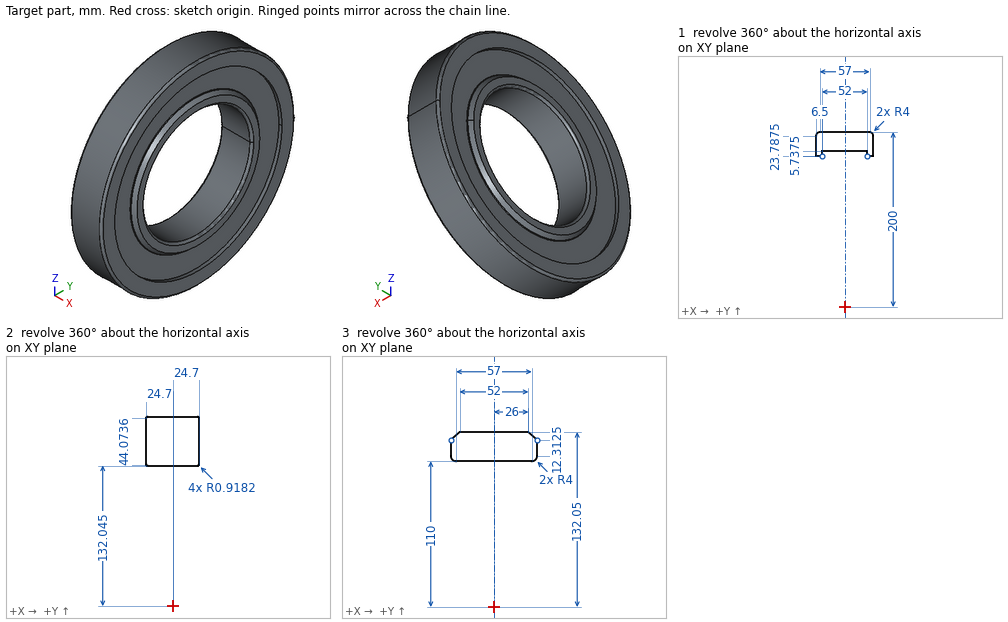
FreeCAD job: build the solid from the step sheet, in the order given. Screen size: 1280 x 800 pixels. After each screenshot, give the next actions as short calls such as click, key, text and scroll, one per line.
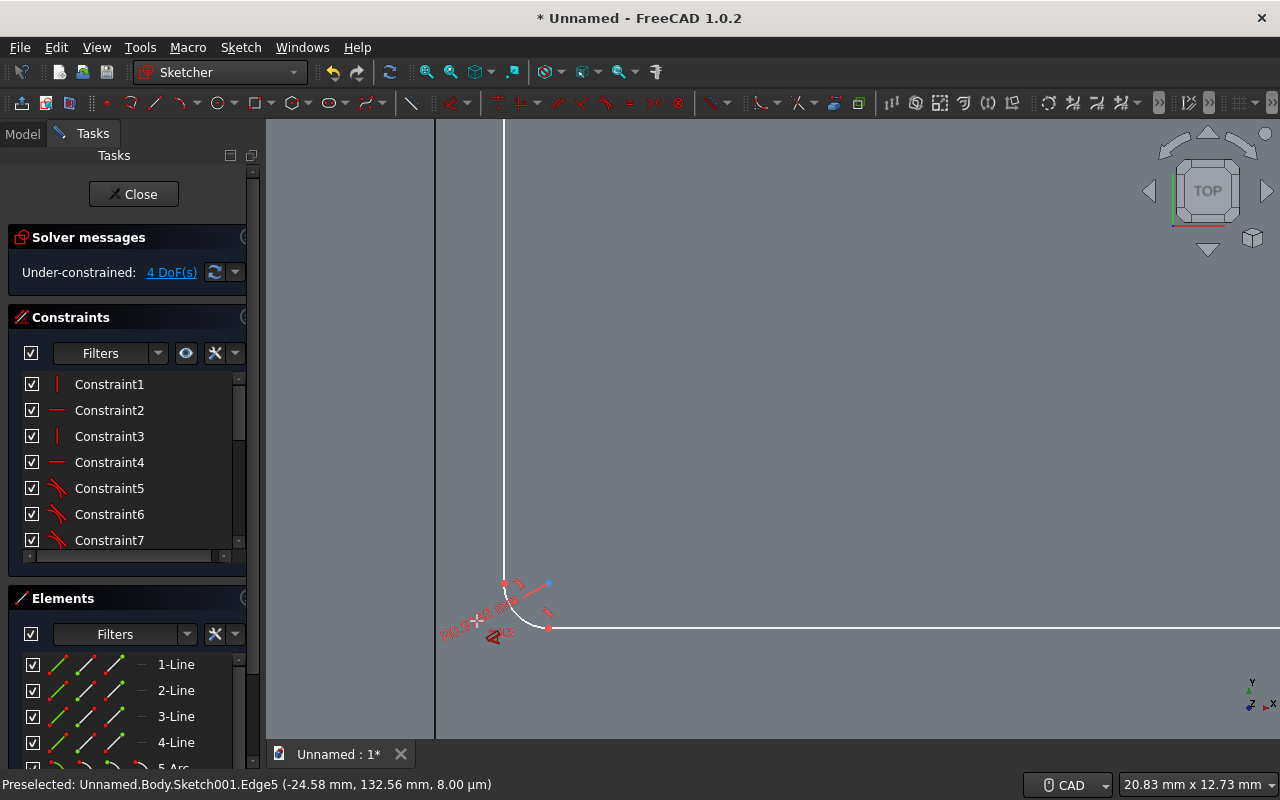
scroll(507, 611, down, 9)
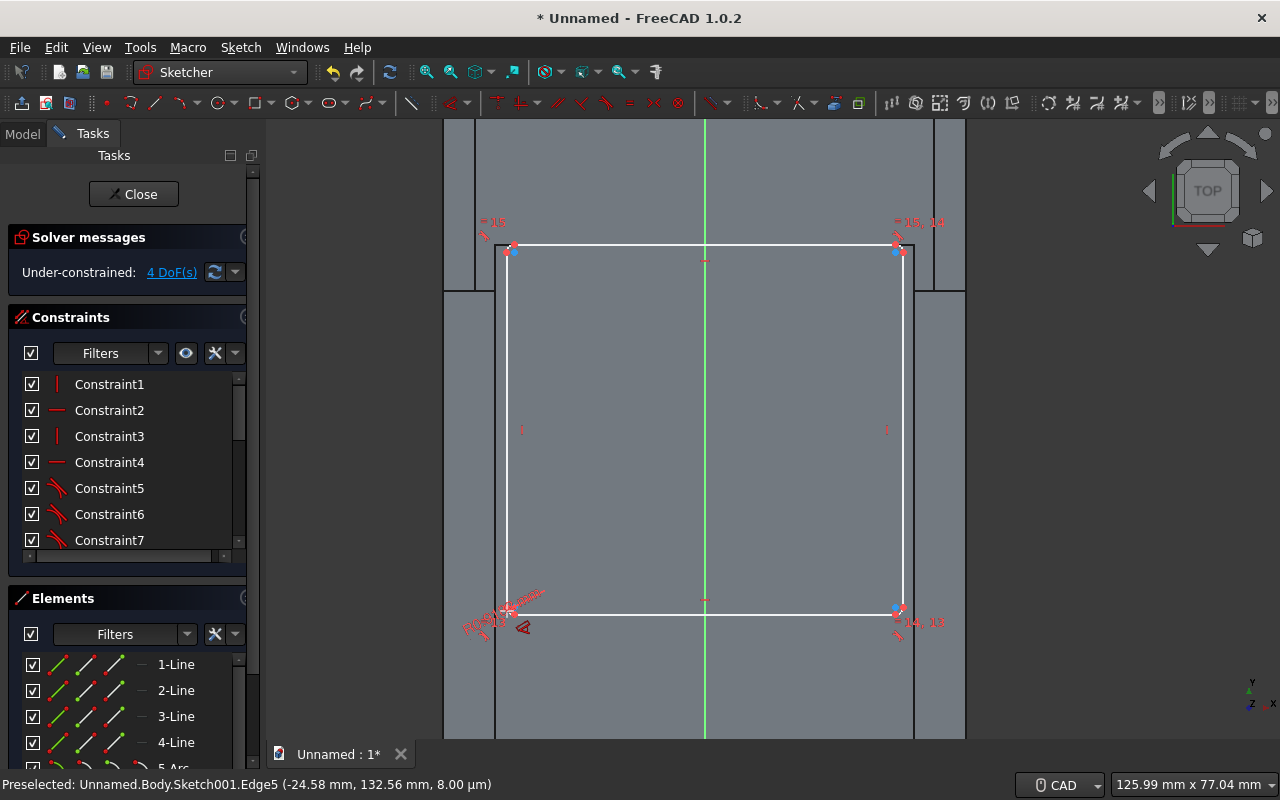
scroll(507, 252, up, 3)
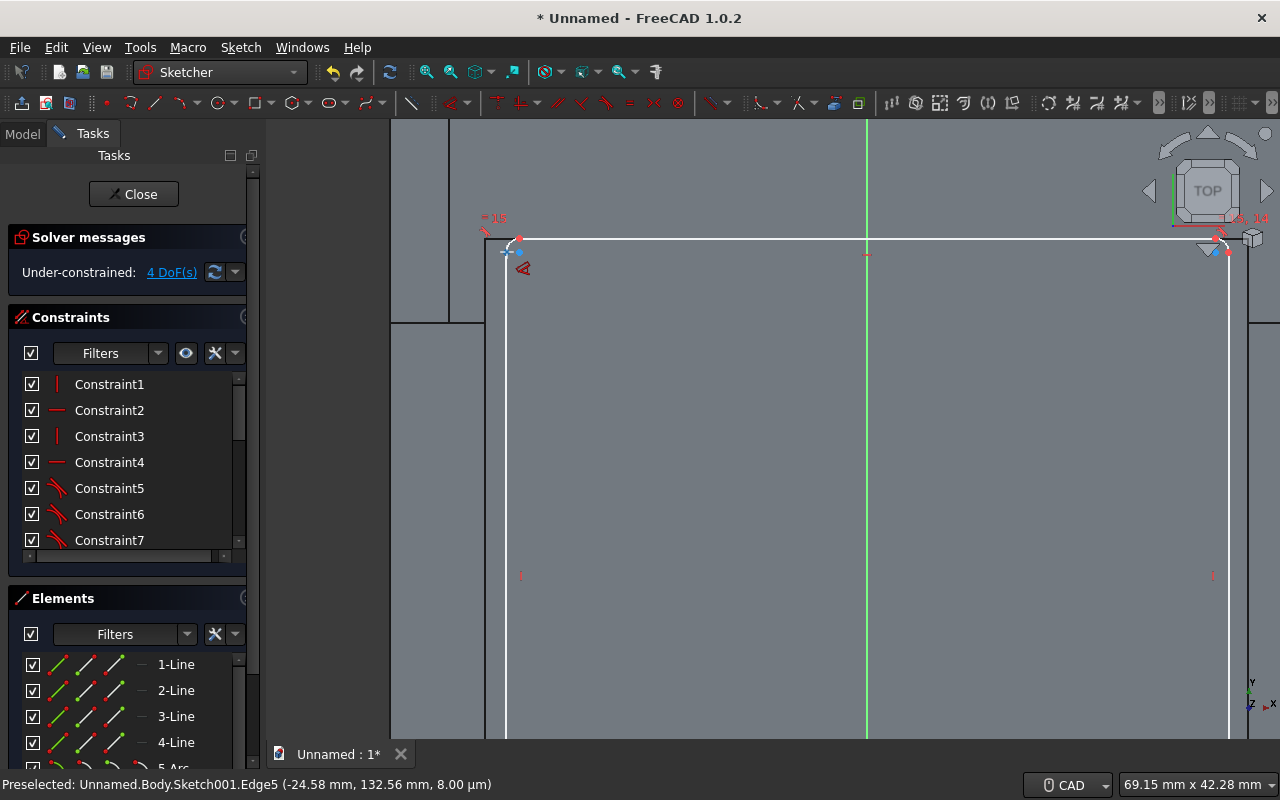
click(506, 252)
click(686, 218)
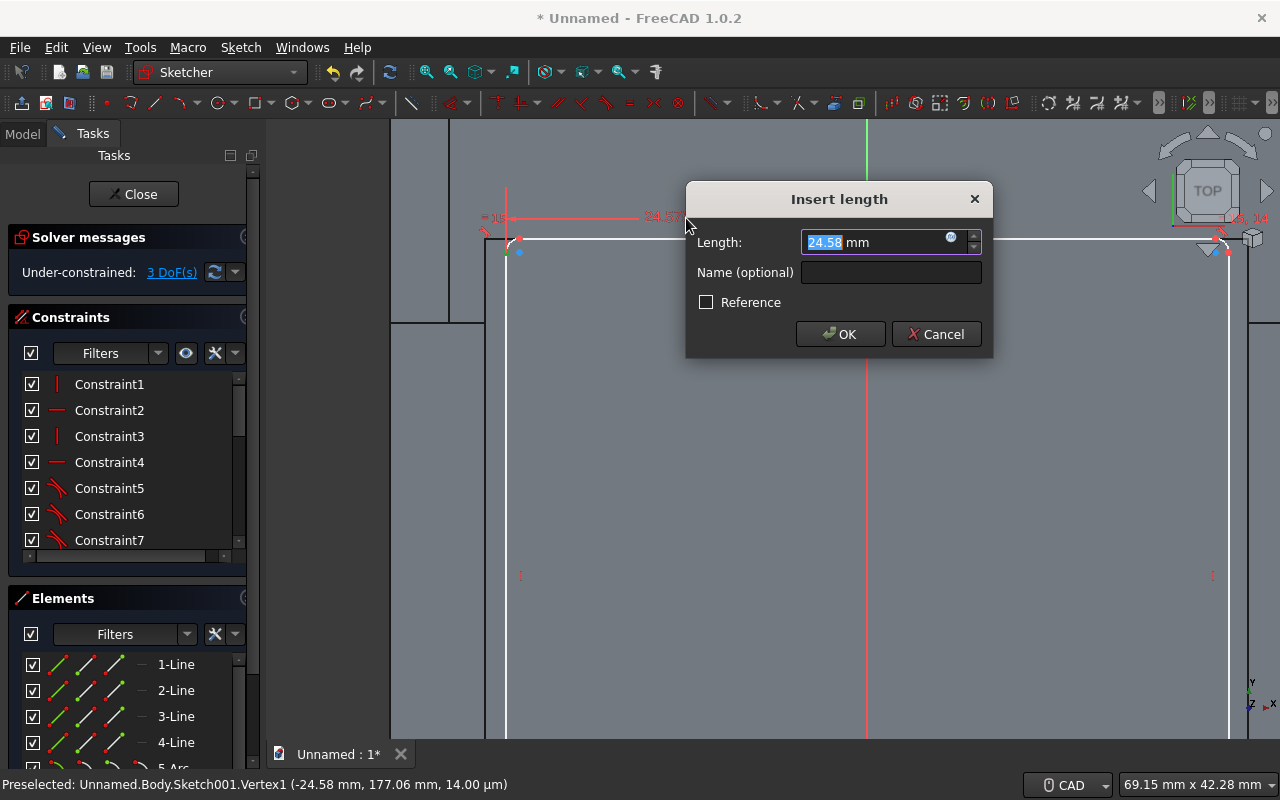
text(24.7)
key(Return)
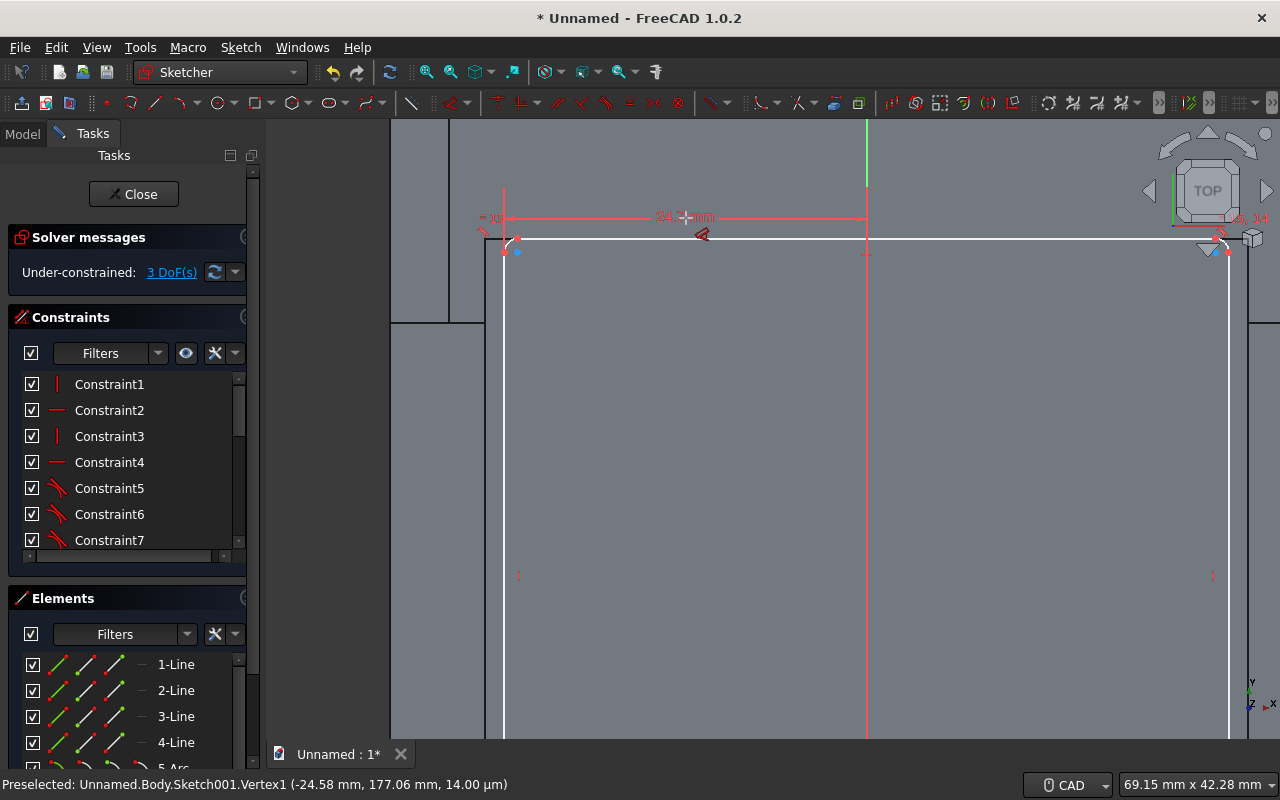
scroll(507, 251, down, 3)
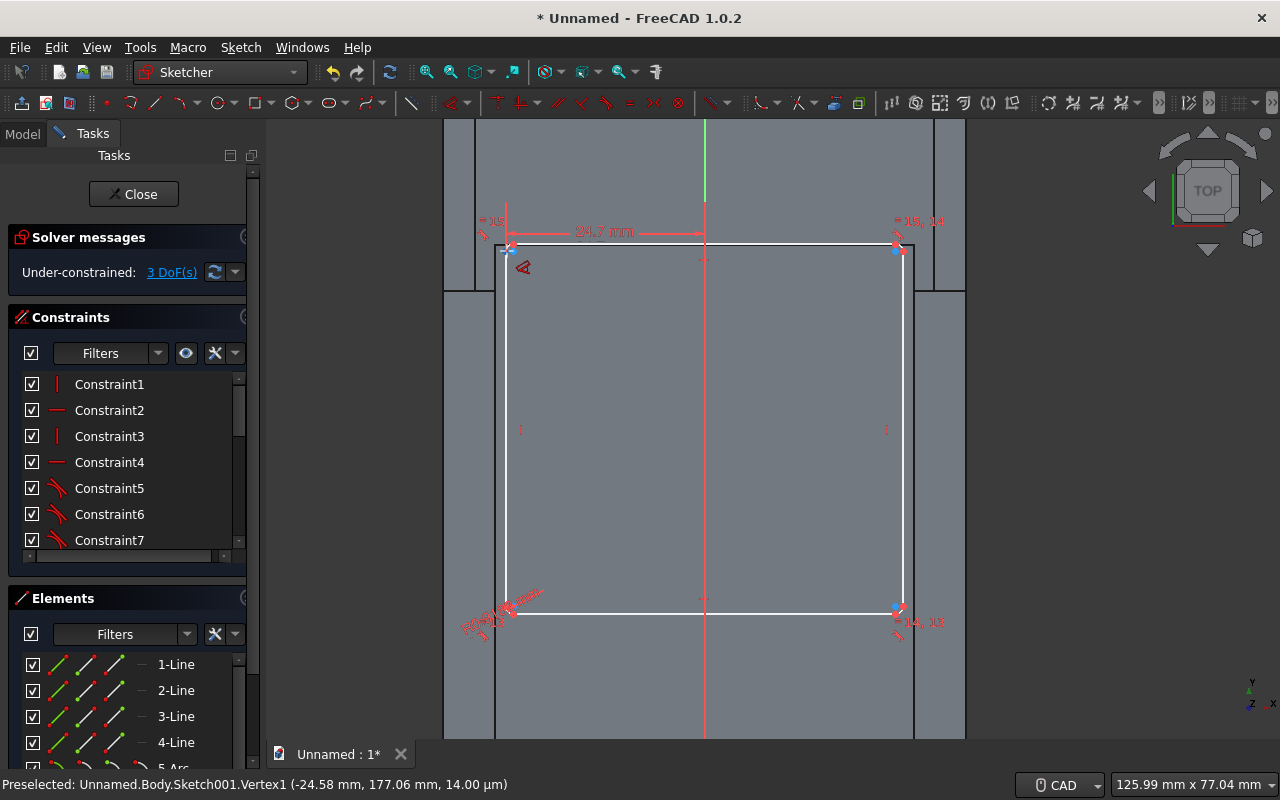
scroll(903, 607, up, 3)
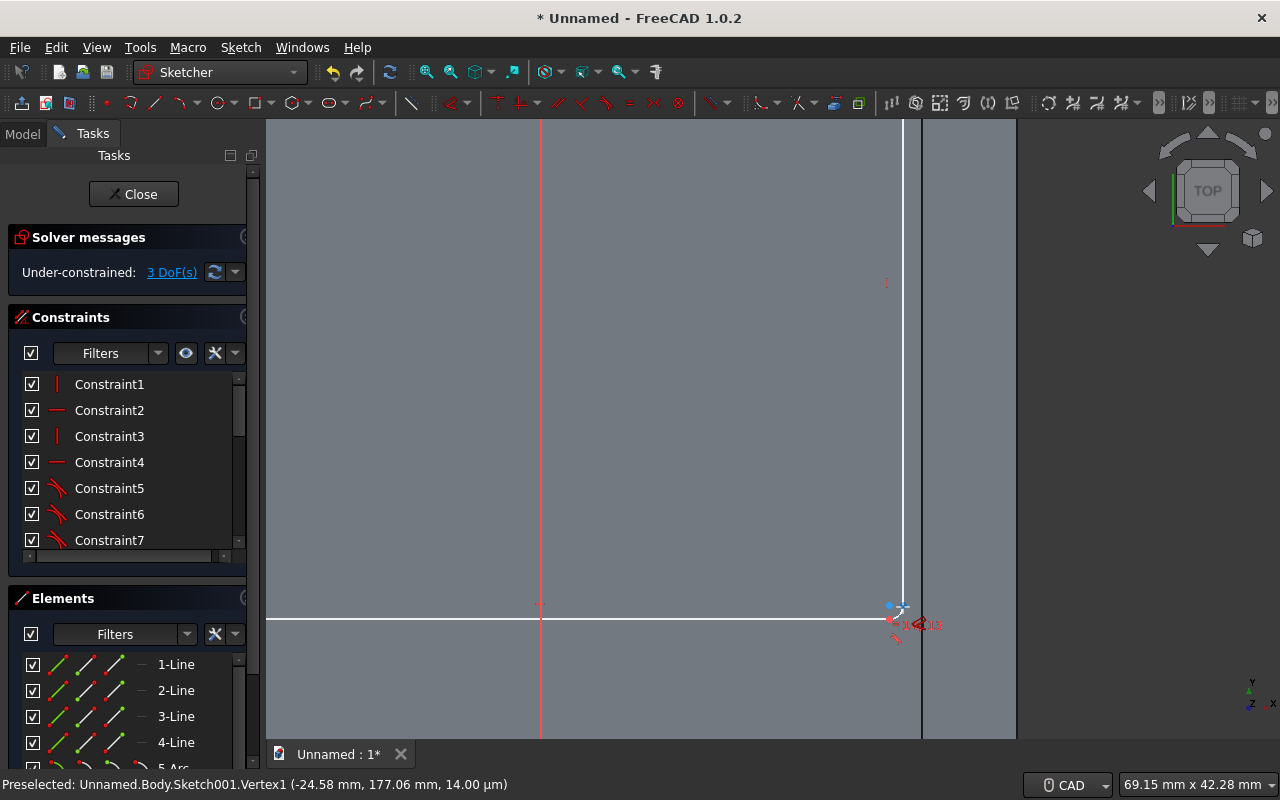
click(903, 606)
click(722, 572)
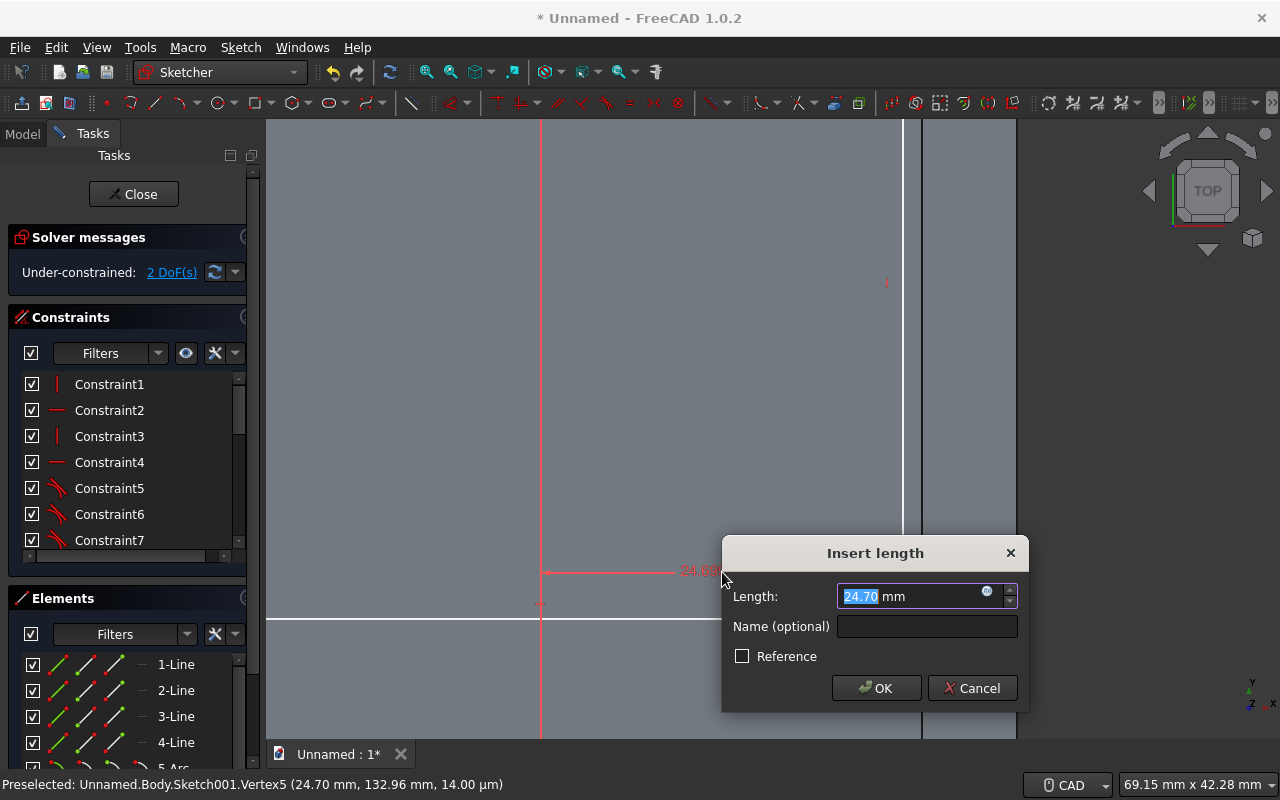
text(24.7)
key(Return)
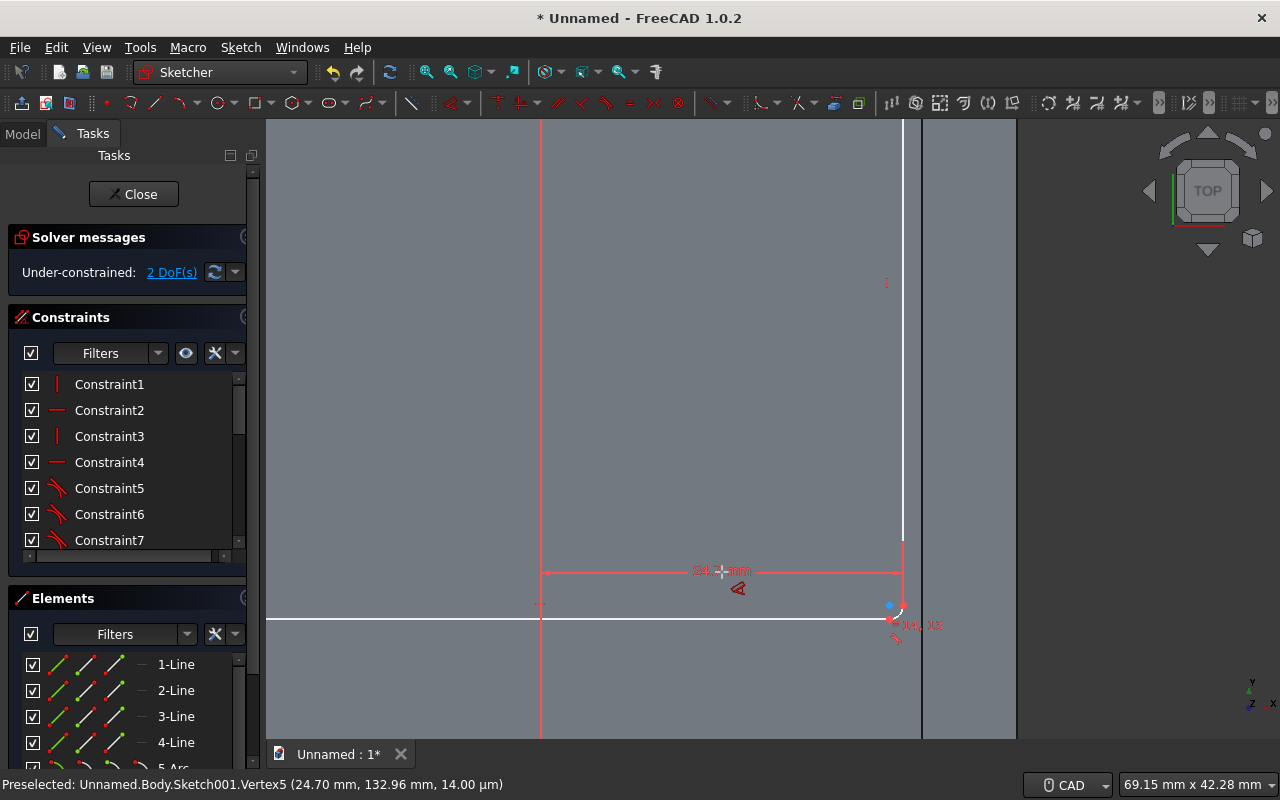
scroll(904, 607, down, 3)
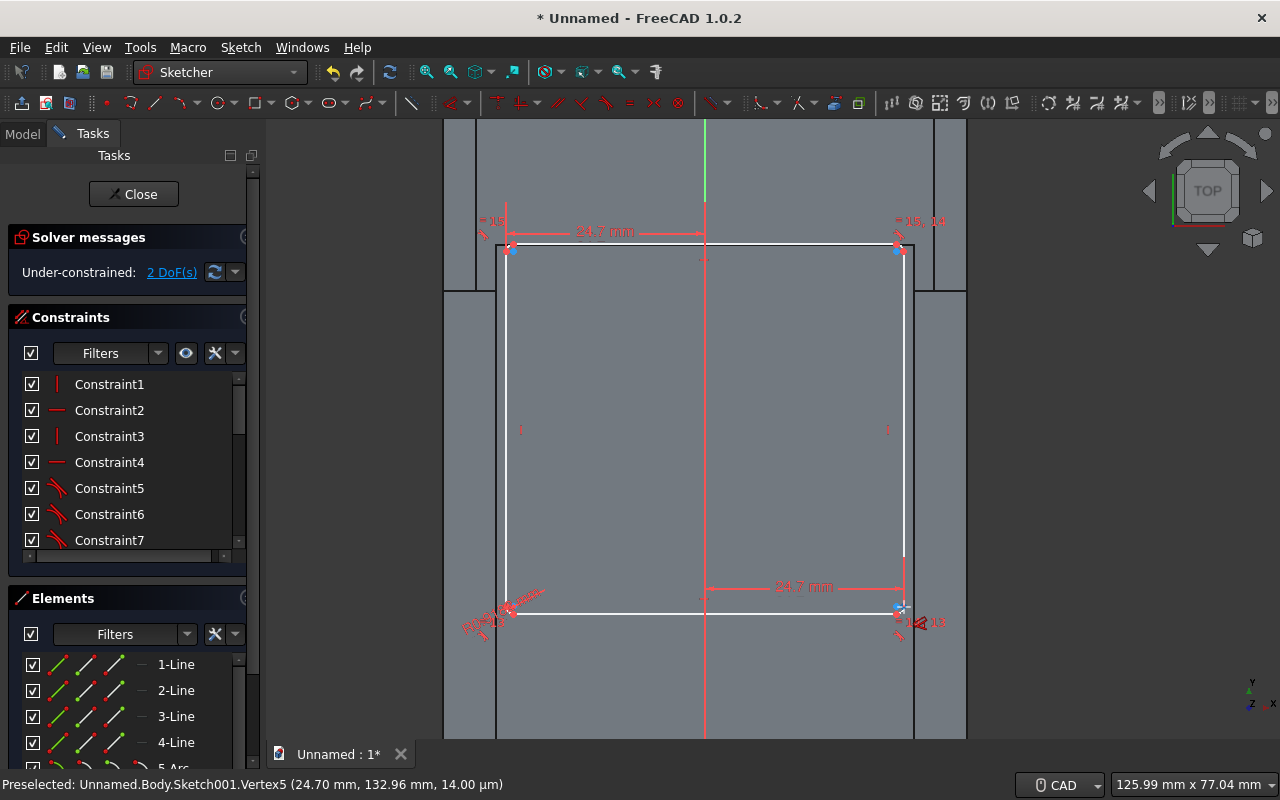
click(506, 358)
click(472, 429)